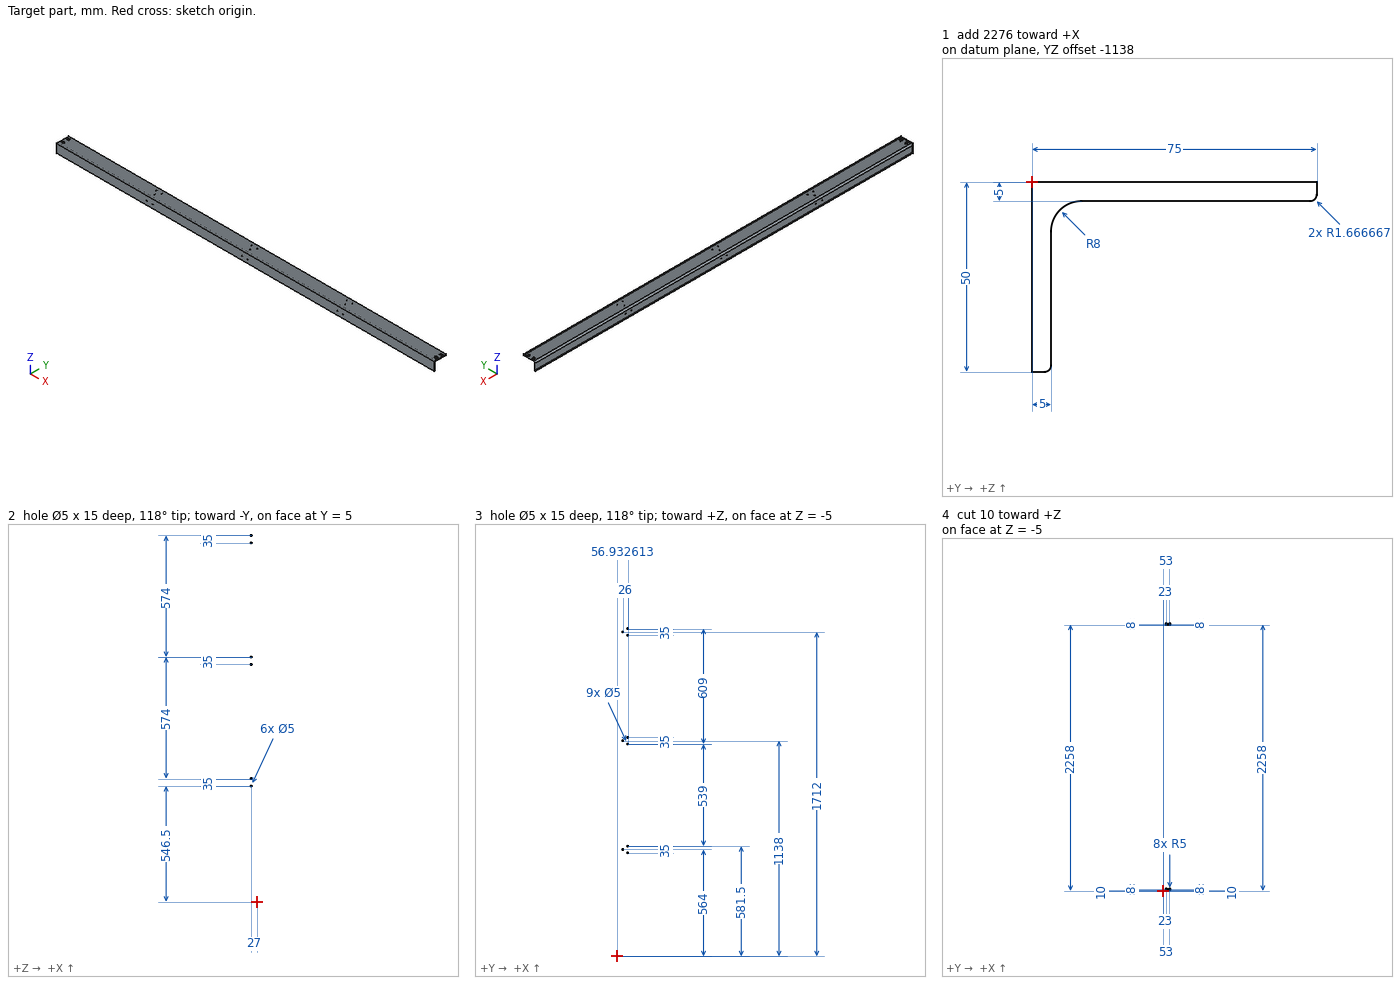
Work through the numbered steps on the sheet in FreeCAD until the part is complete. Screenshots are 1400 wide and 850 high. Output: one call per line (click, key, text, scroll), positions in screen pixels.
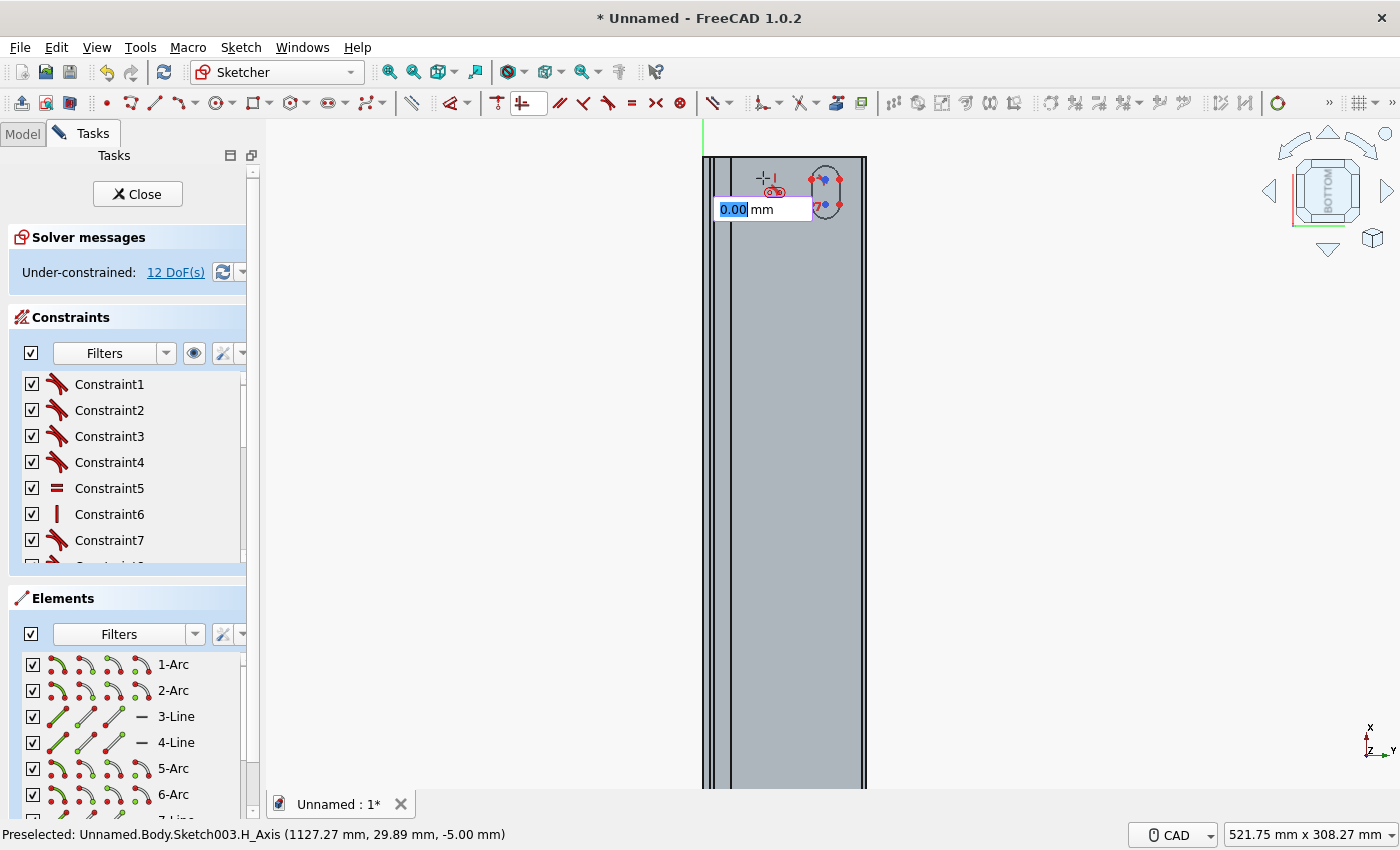
scroll(775, 187, up, 2)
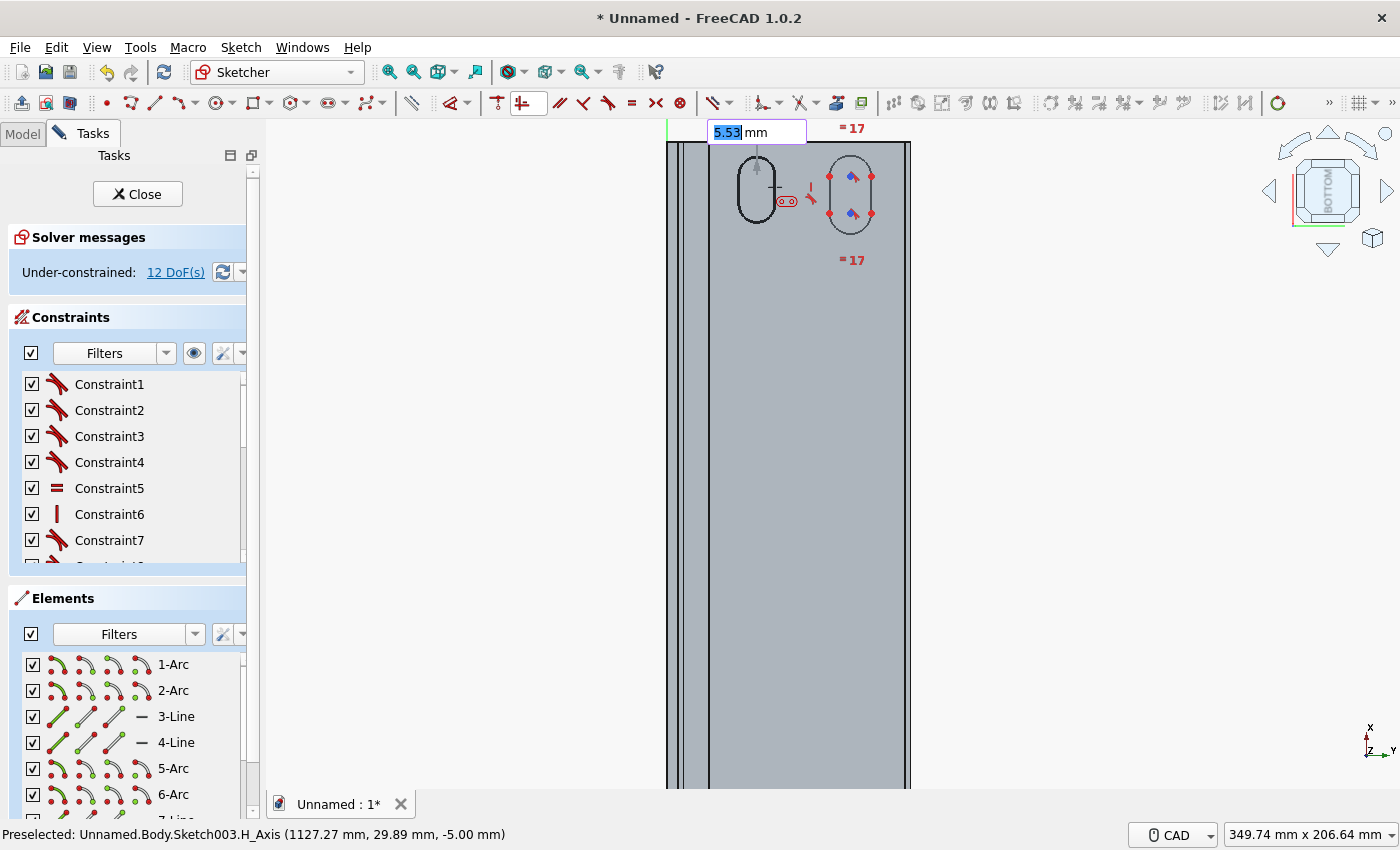
click(774, 187)
key(Escape)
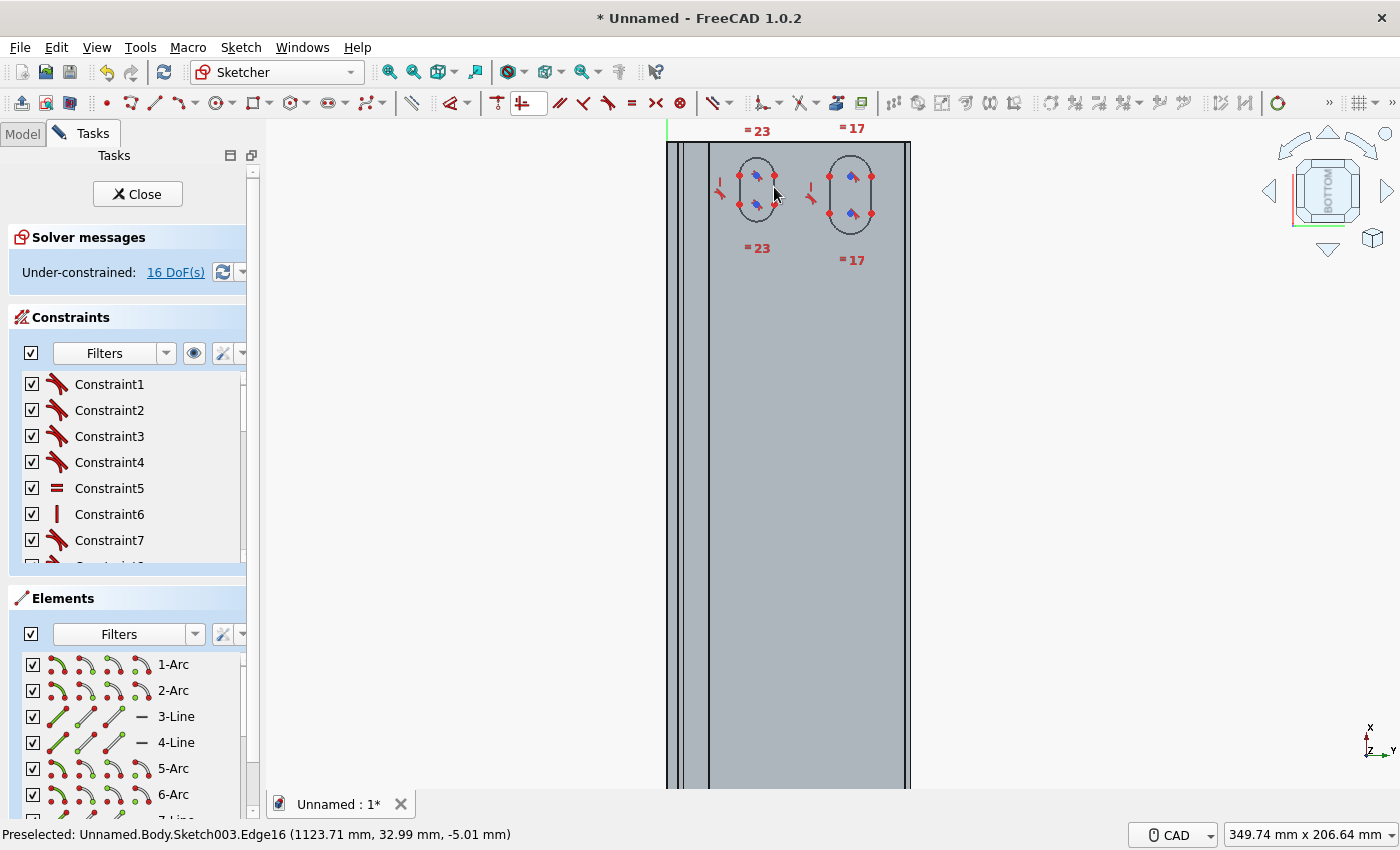
scroll(764, 235, down, 14)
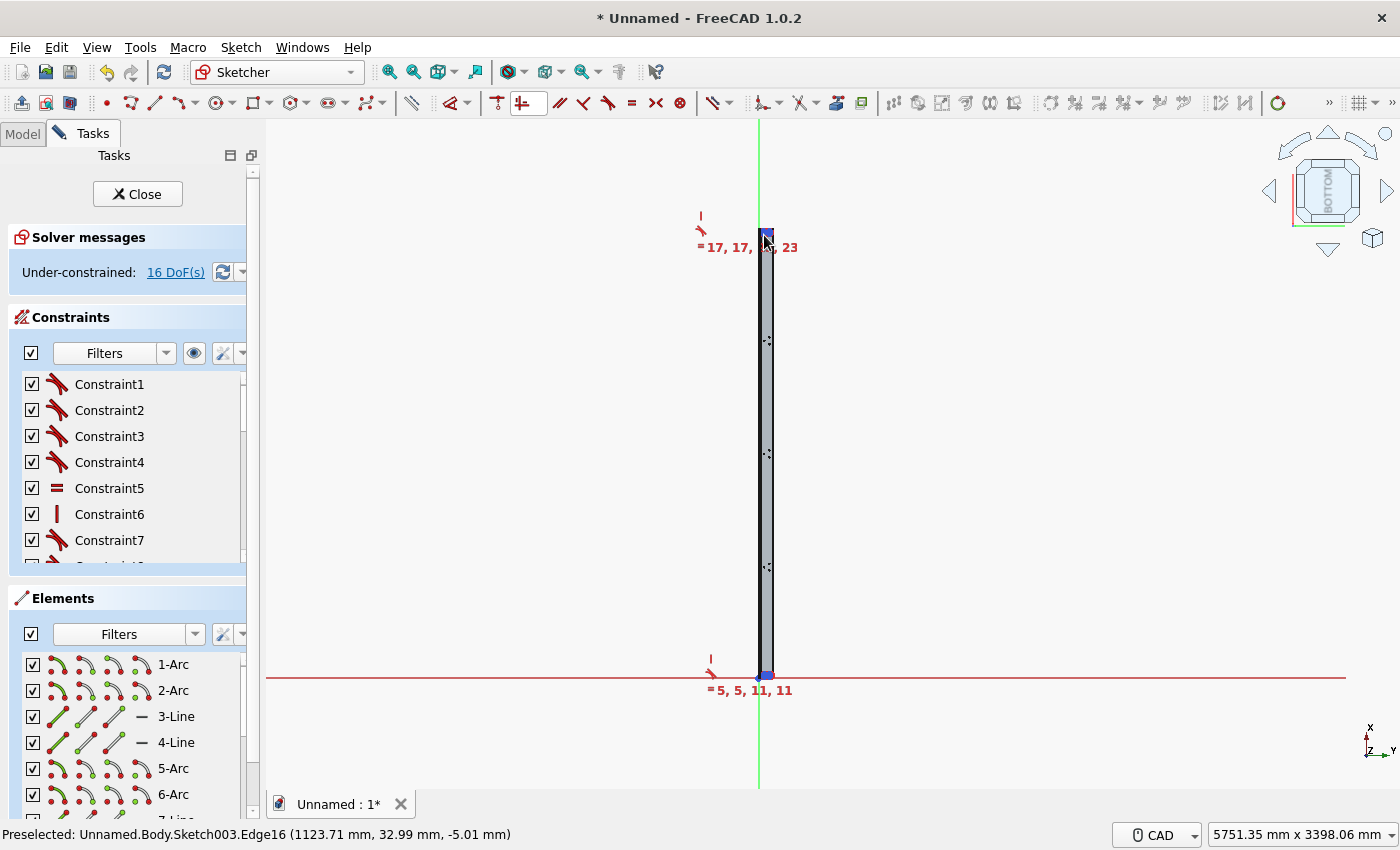
scroll(769, 677, up, 14)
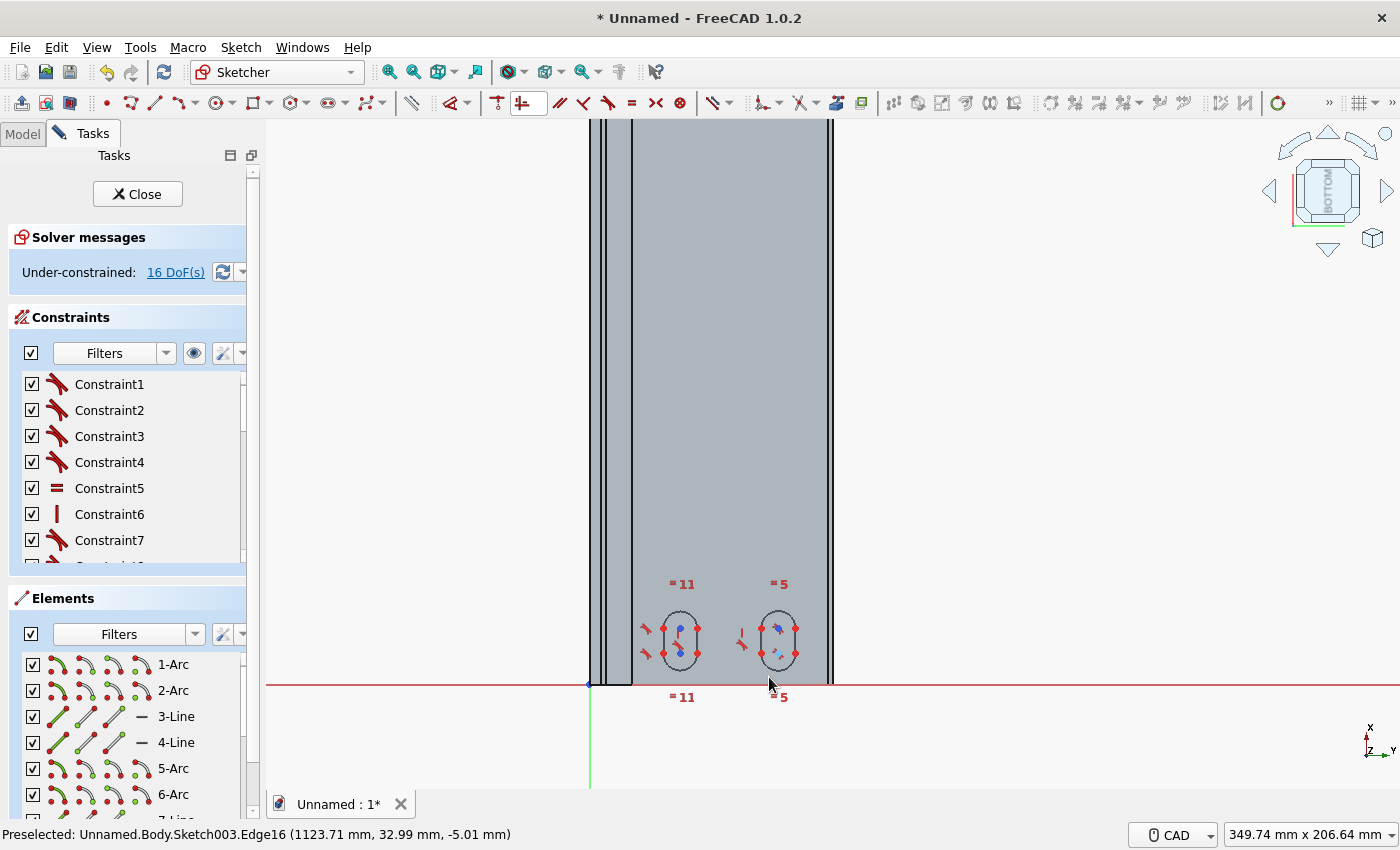
click(768, 667)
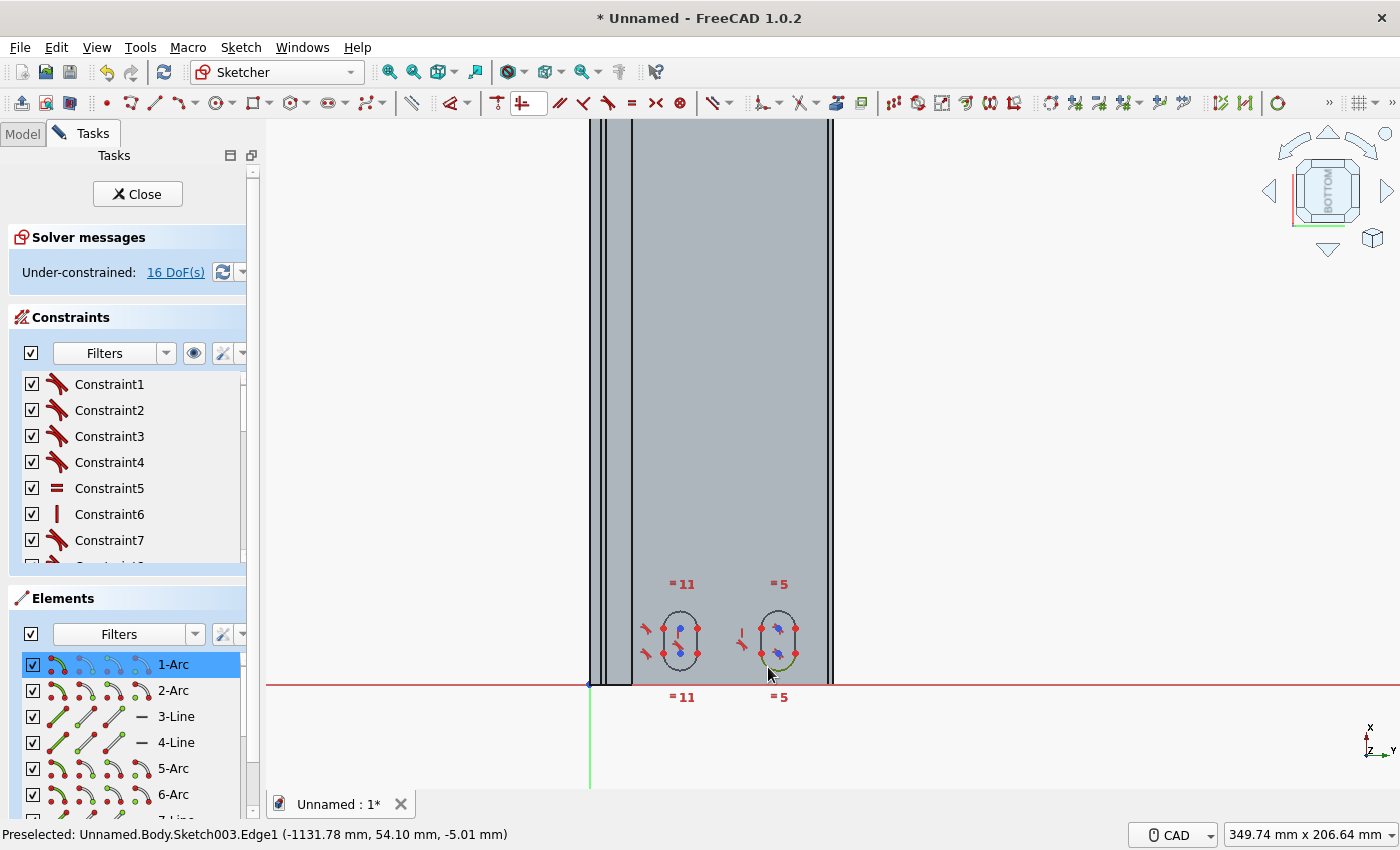
click(671, 667)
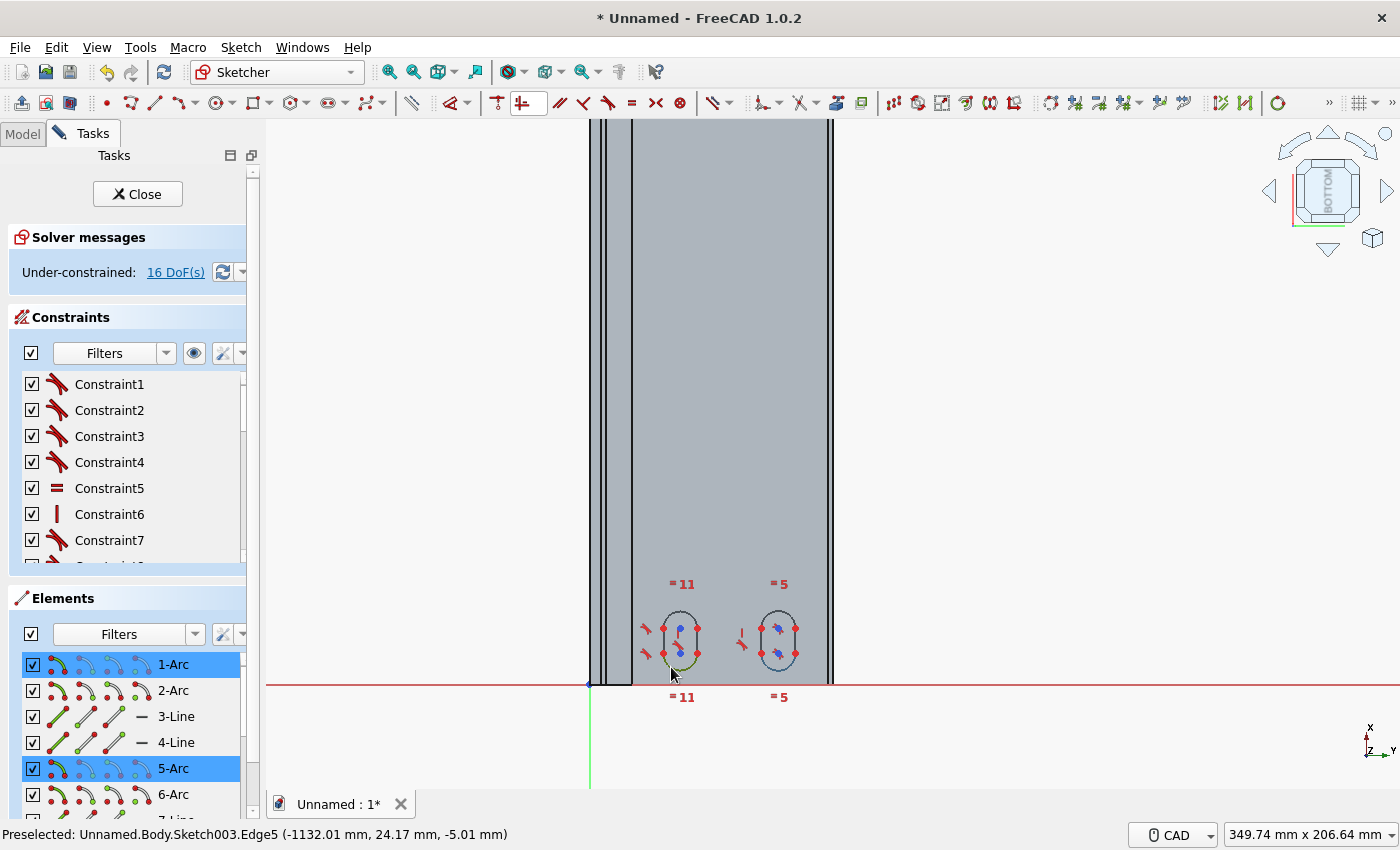
scroll(769, 677, down, 14)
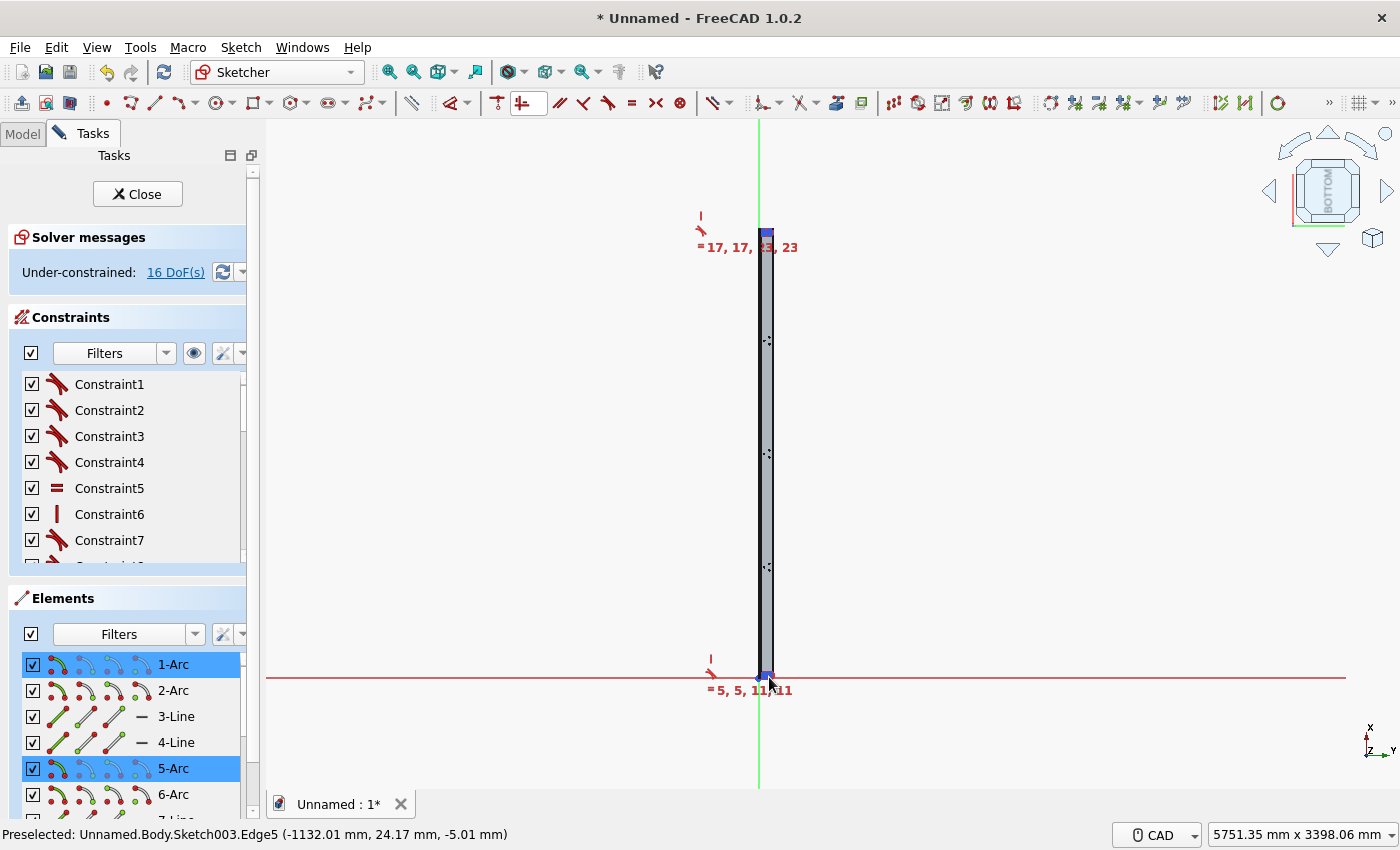
scroll(769, 235, up, 13)